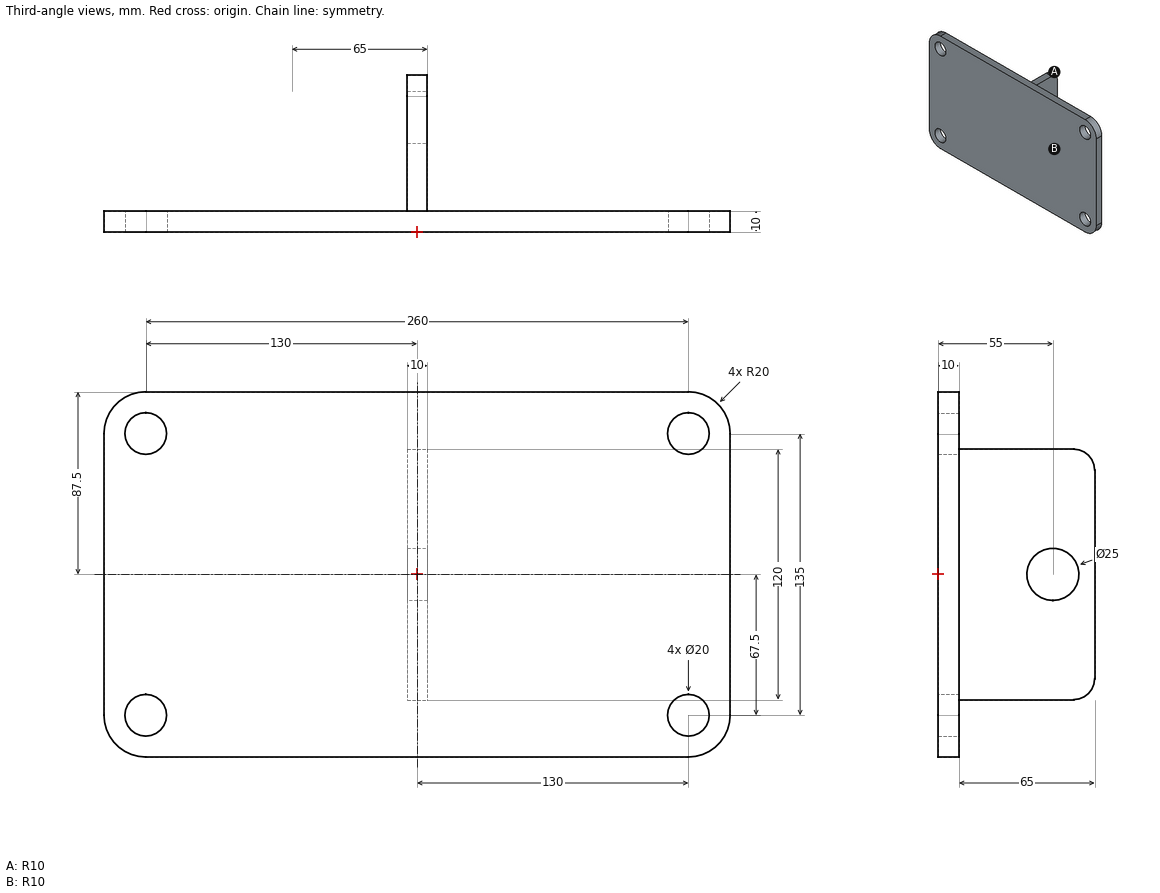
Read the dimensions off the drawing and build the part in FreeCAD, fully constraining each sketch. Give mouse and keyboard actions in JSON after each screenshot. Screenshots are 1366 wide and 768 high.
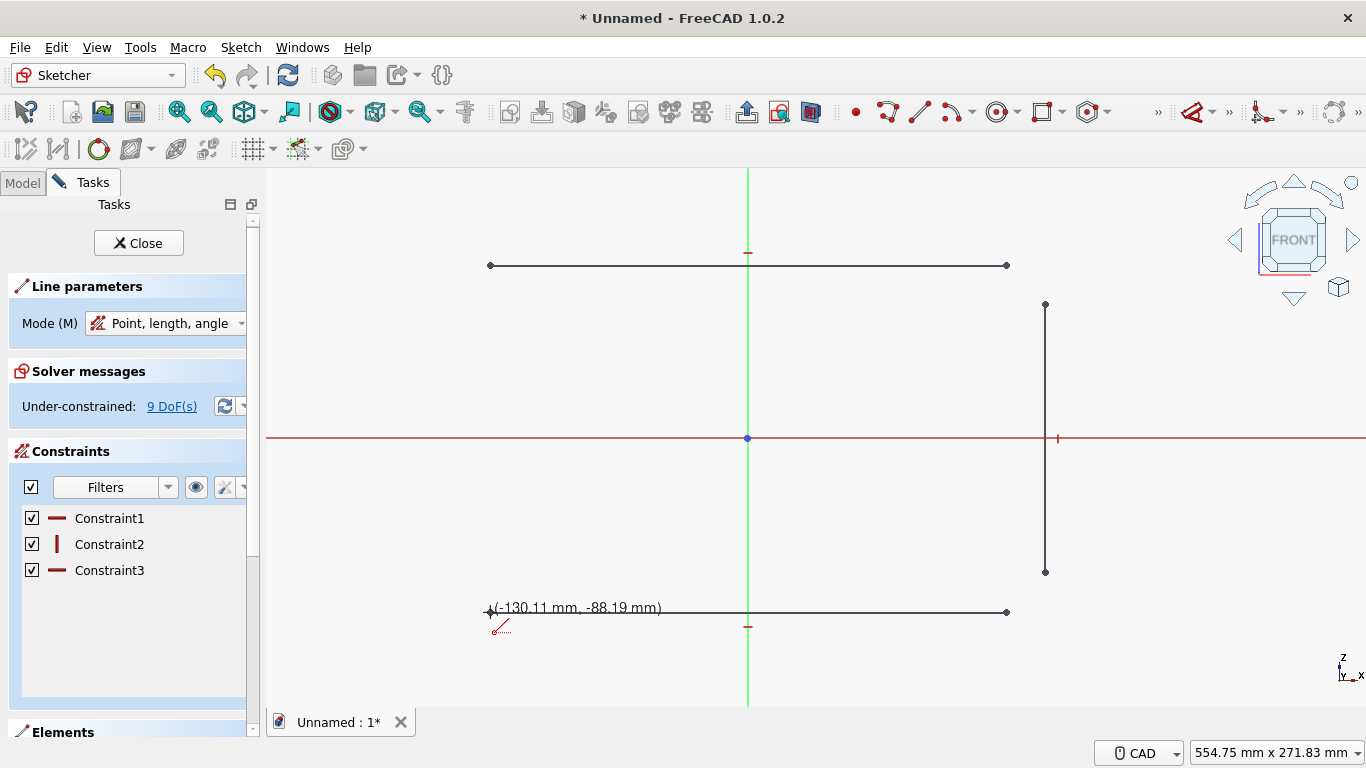
{"action": "left_click", "coordinate": [451, 572]}
{"action": "left_click", "coordinate": [451, 304]}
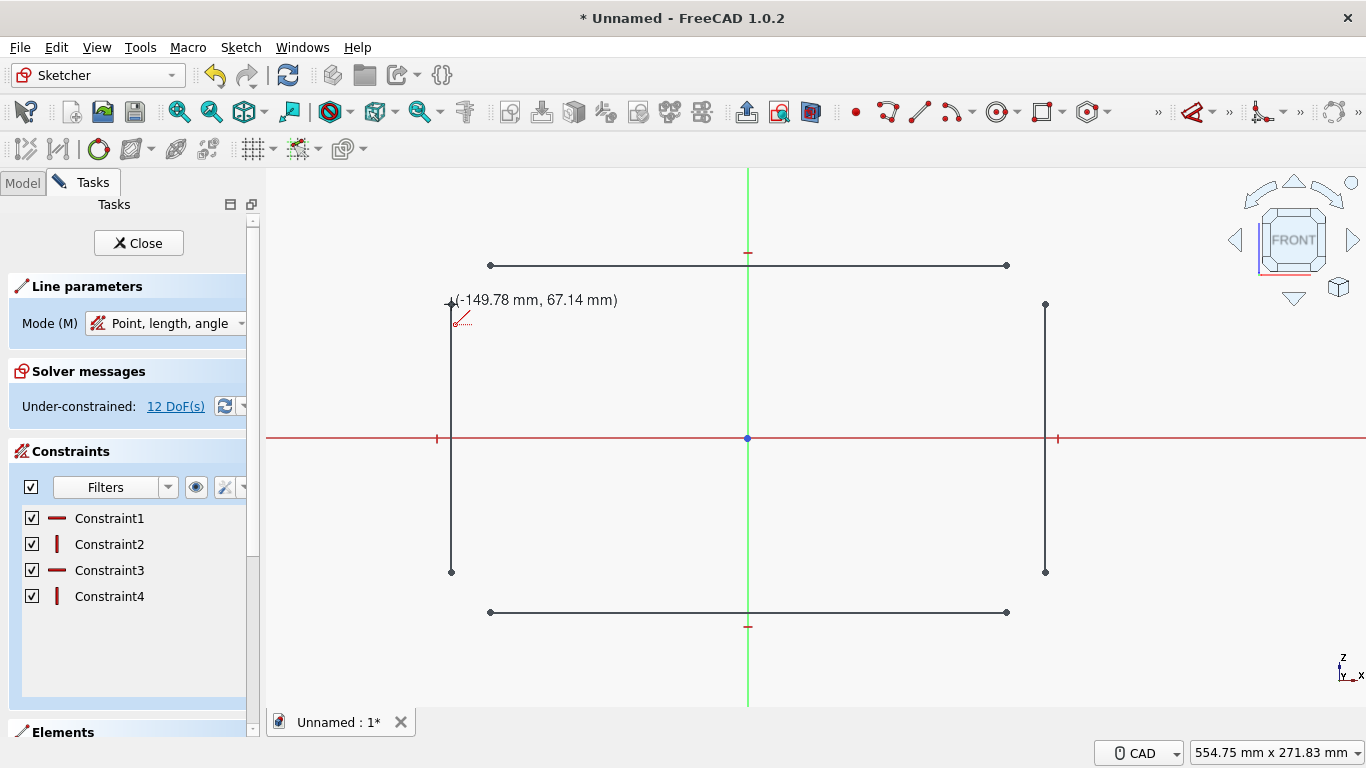
{"action": "key", "text": "g 3 a"}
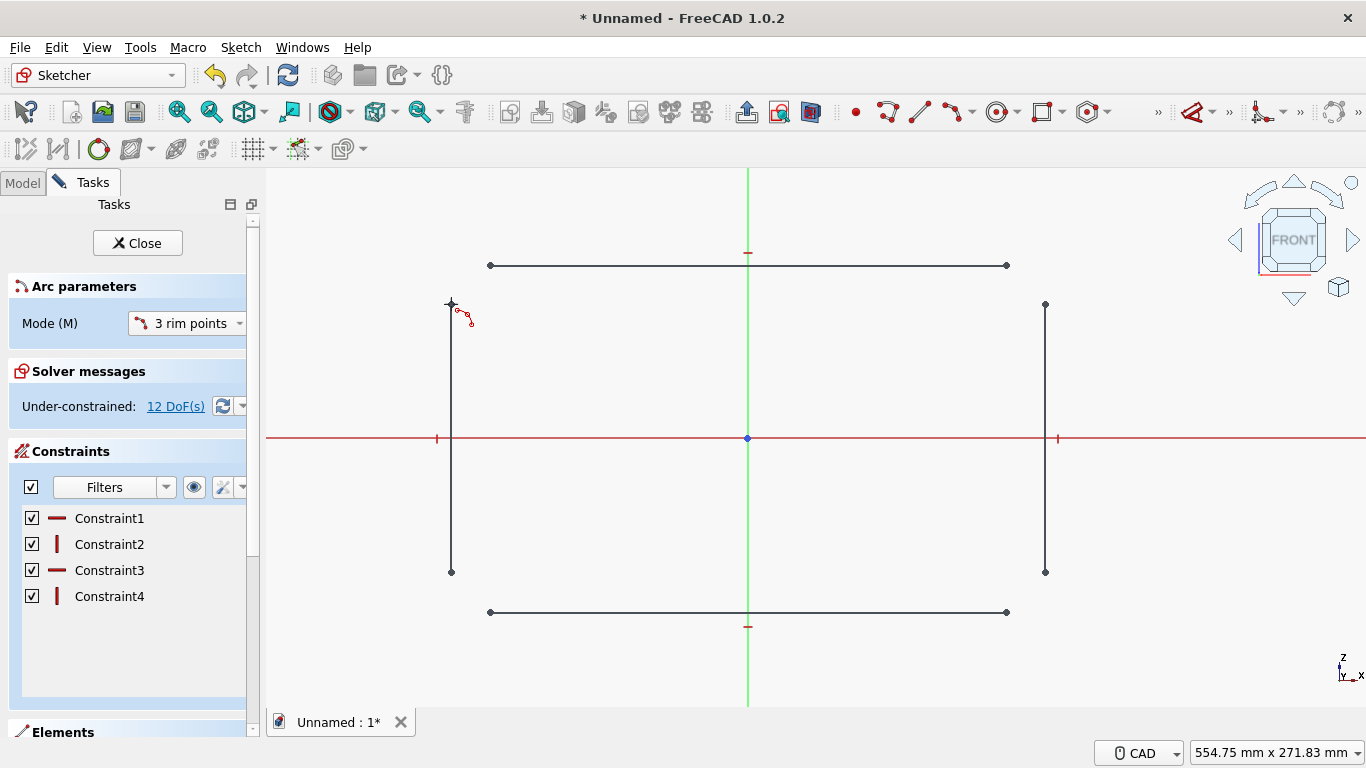
{"action": "left_click", "coordinate": [1006, 266]}
{"action": "left_click", "coordinate": [1045, 305]}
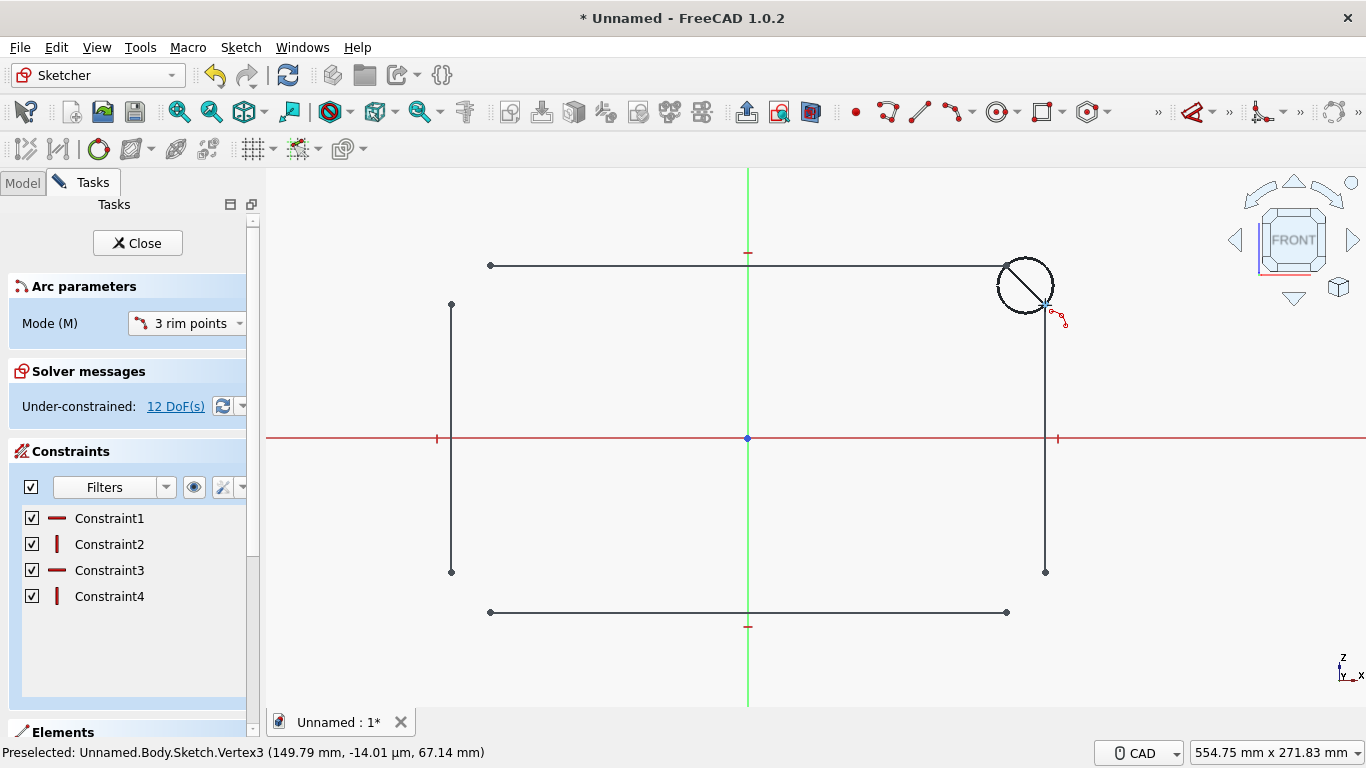
{"action": "scroll", "coordinate": [1034, 276], "scroll_direction": "up", "scroll_amount": 2}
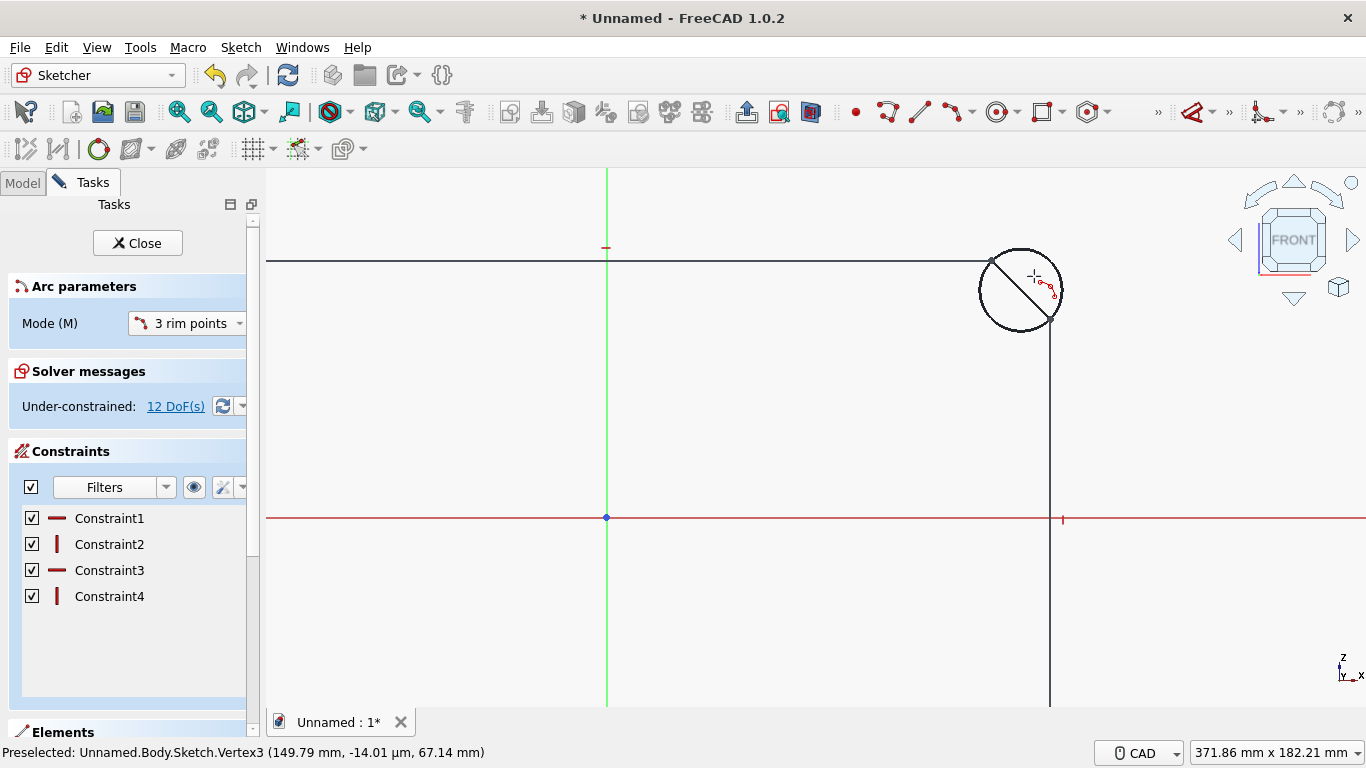
{"action": "left_click", "coordinate": [1033, 276]}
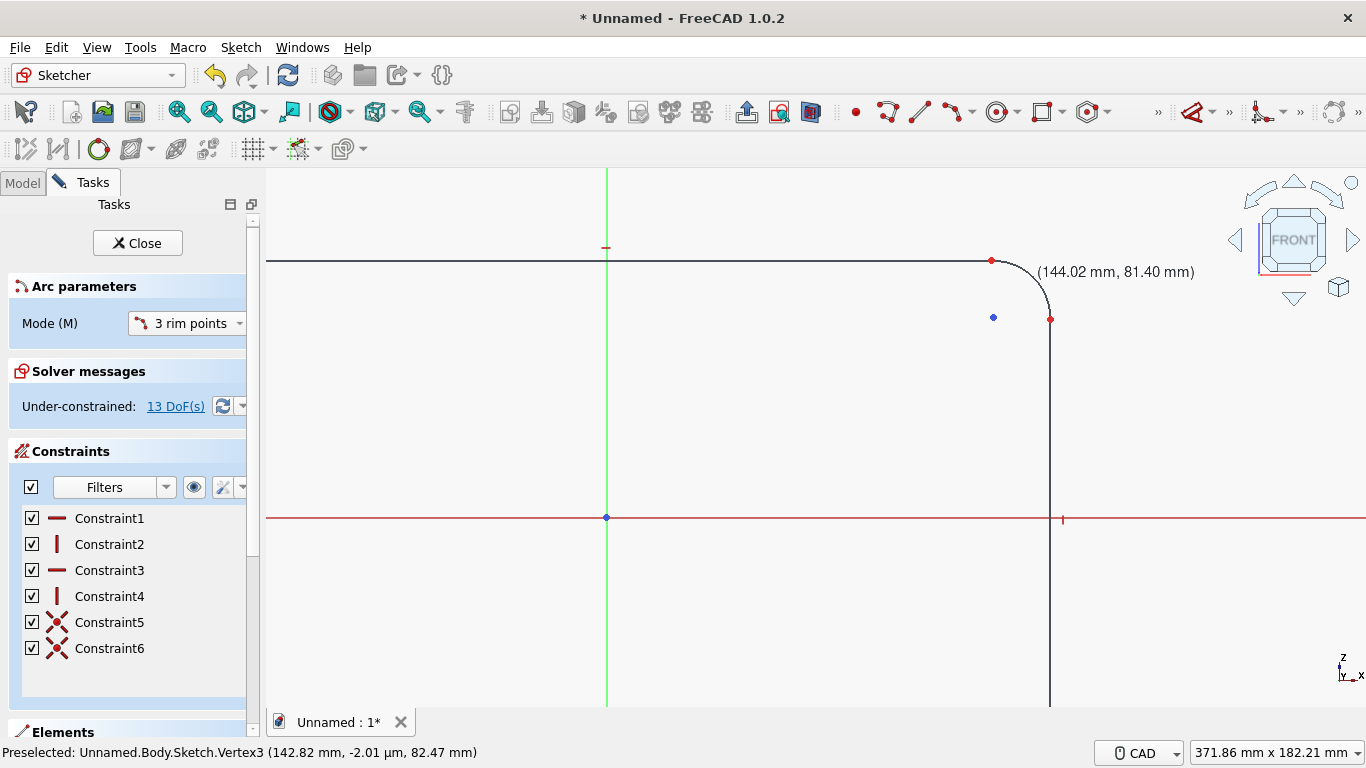
{"action": "scroll", "coordinate": [1033, 274], "scroll_direction": "down", "scroll_amount": 2}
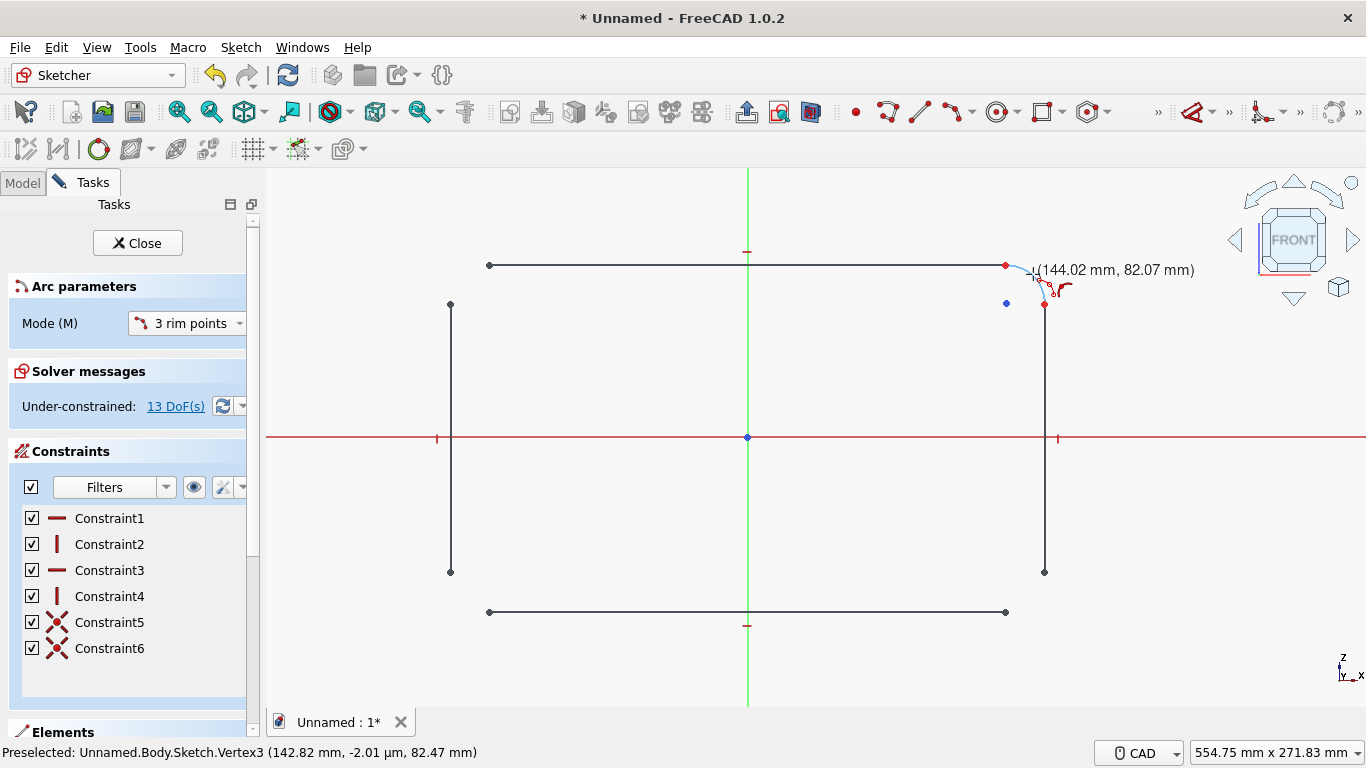
{"action": "left_click", "coordinate": [1045, 572]}
{"action": "left_click", "coordinate": [1006, 612]}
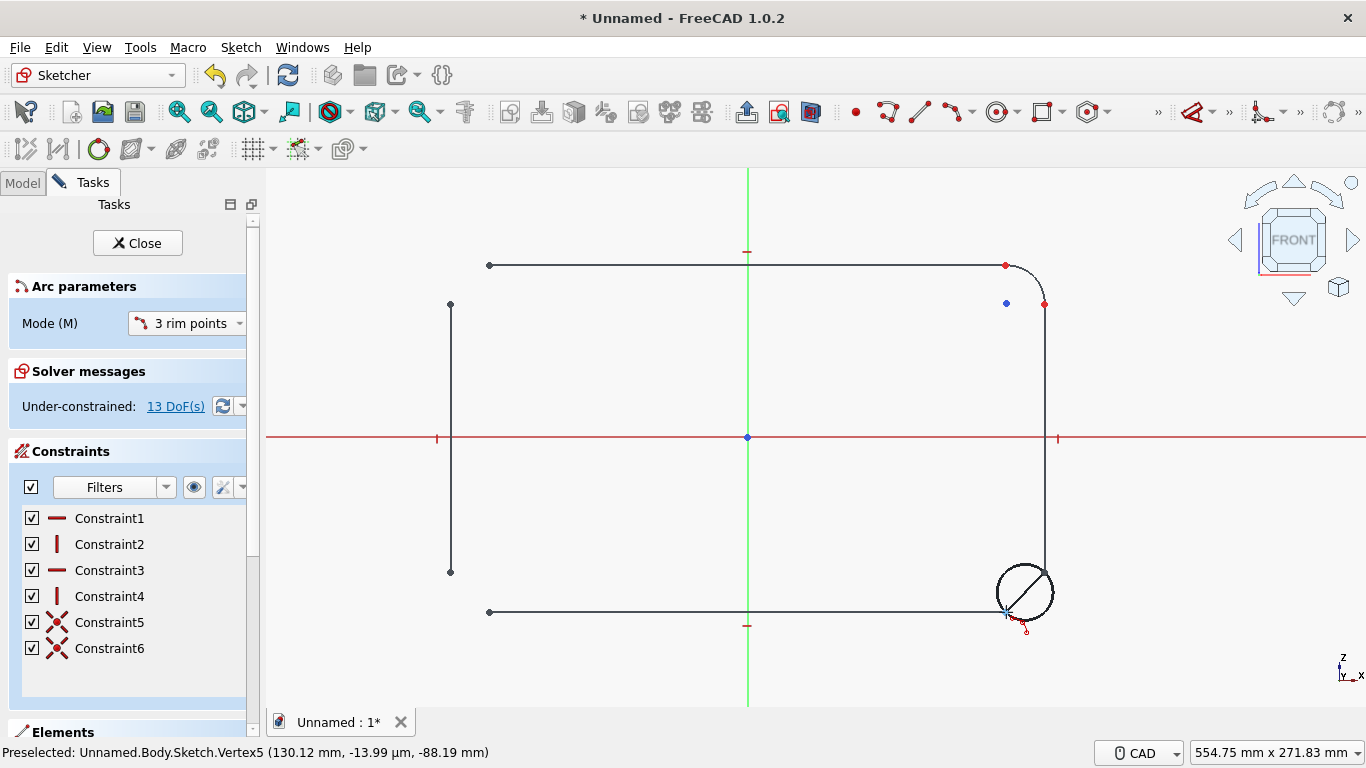
{"action": "scroll", "coordinate": [1033, 599], "scroll_direction": "up", "scroll_amount": 2}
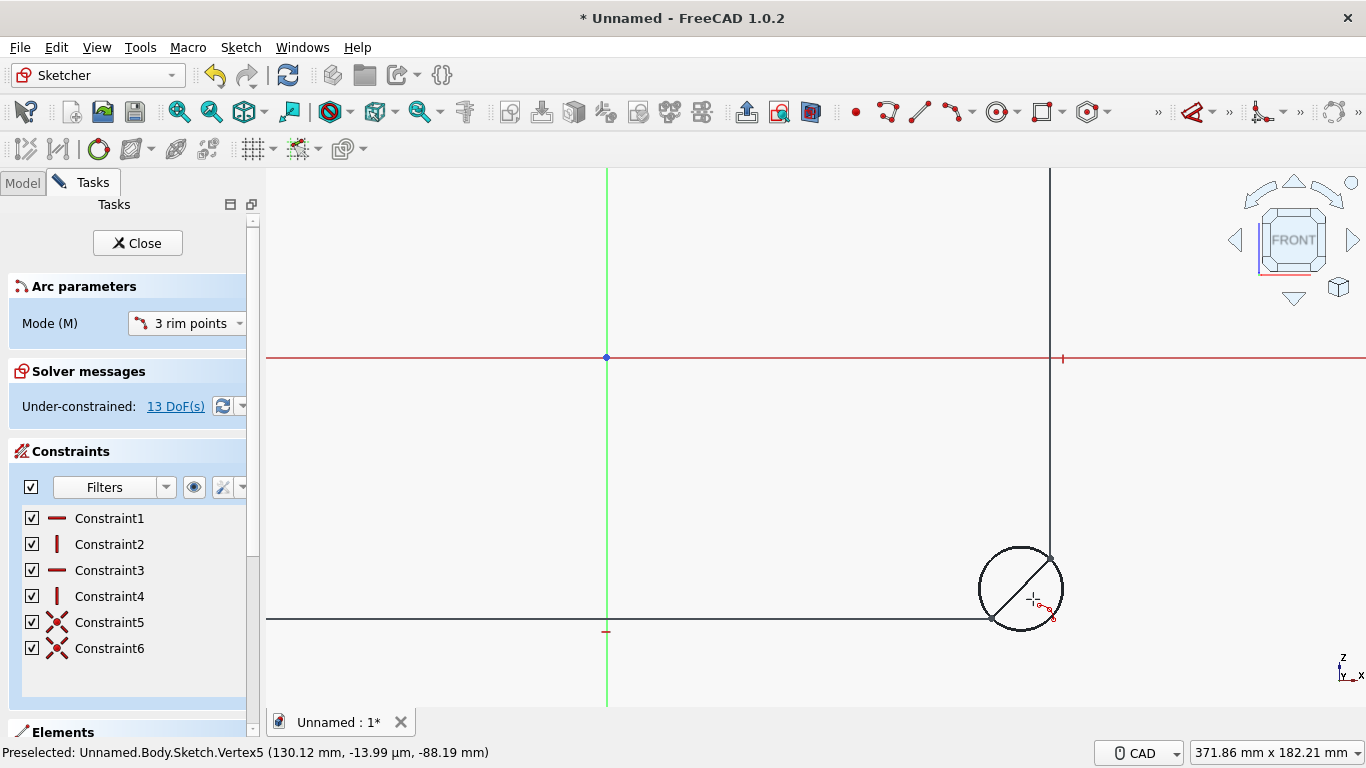
{"action": "left_click", "coordinate": [1033, 599]}